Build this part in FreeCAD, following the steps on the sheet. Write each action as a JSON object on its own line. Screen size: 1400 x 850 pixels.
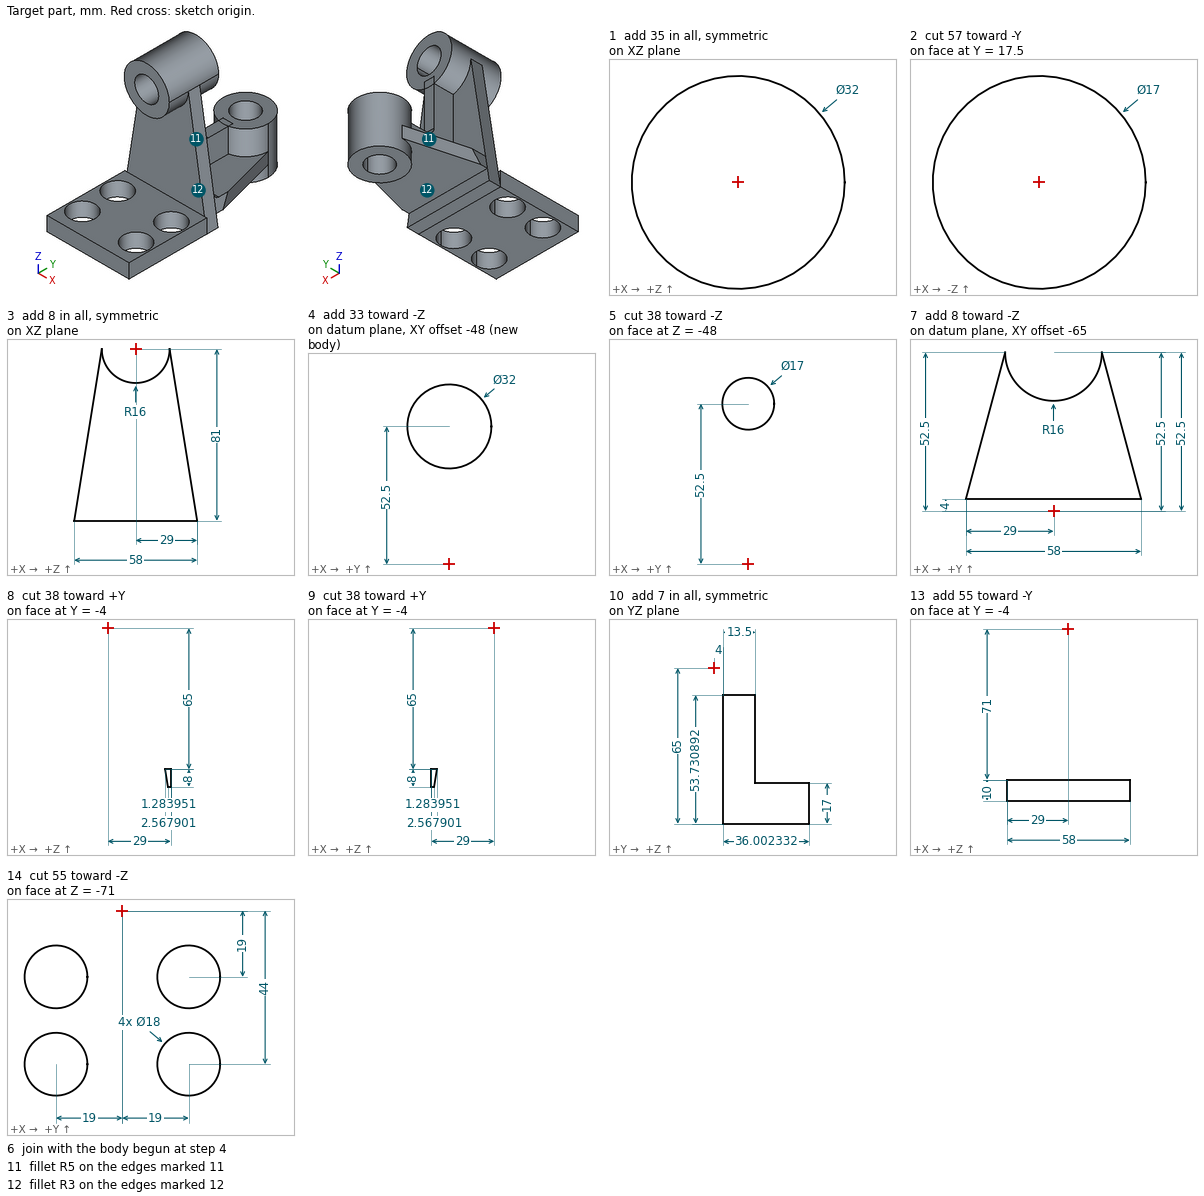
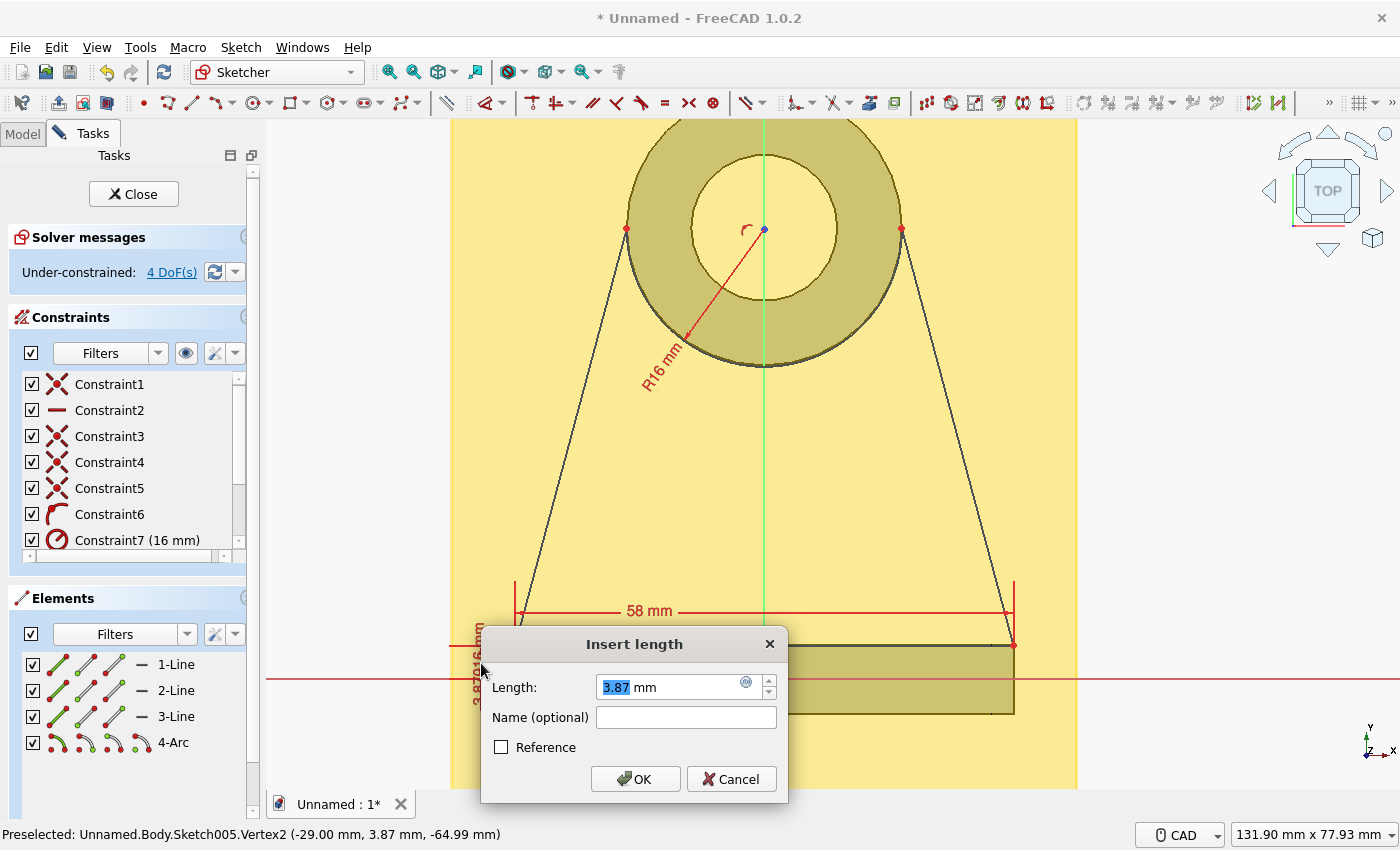
{"action": "type", "text": "4"}
{"action": "key", "text": "Return"}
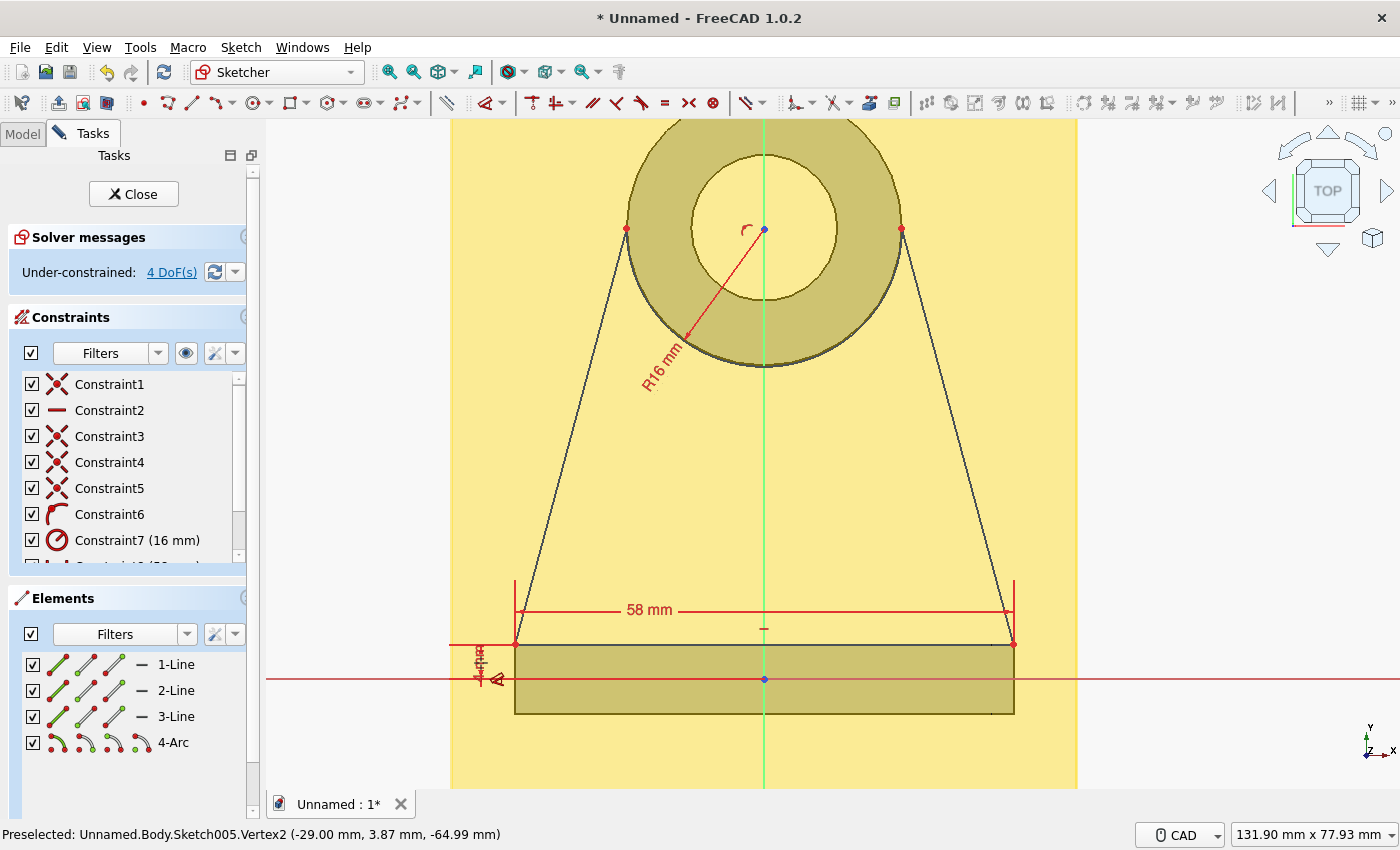
{"action": "left_click", "coordinate": [515, 645]}
{"action": "left_click", "coordinate": [640, 713]}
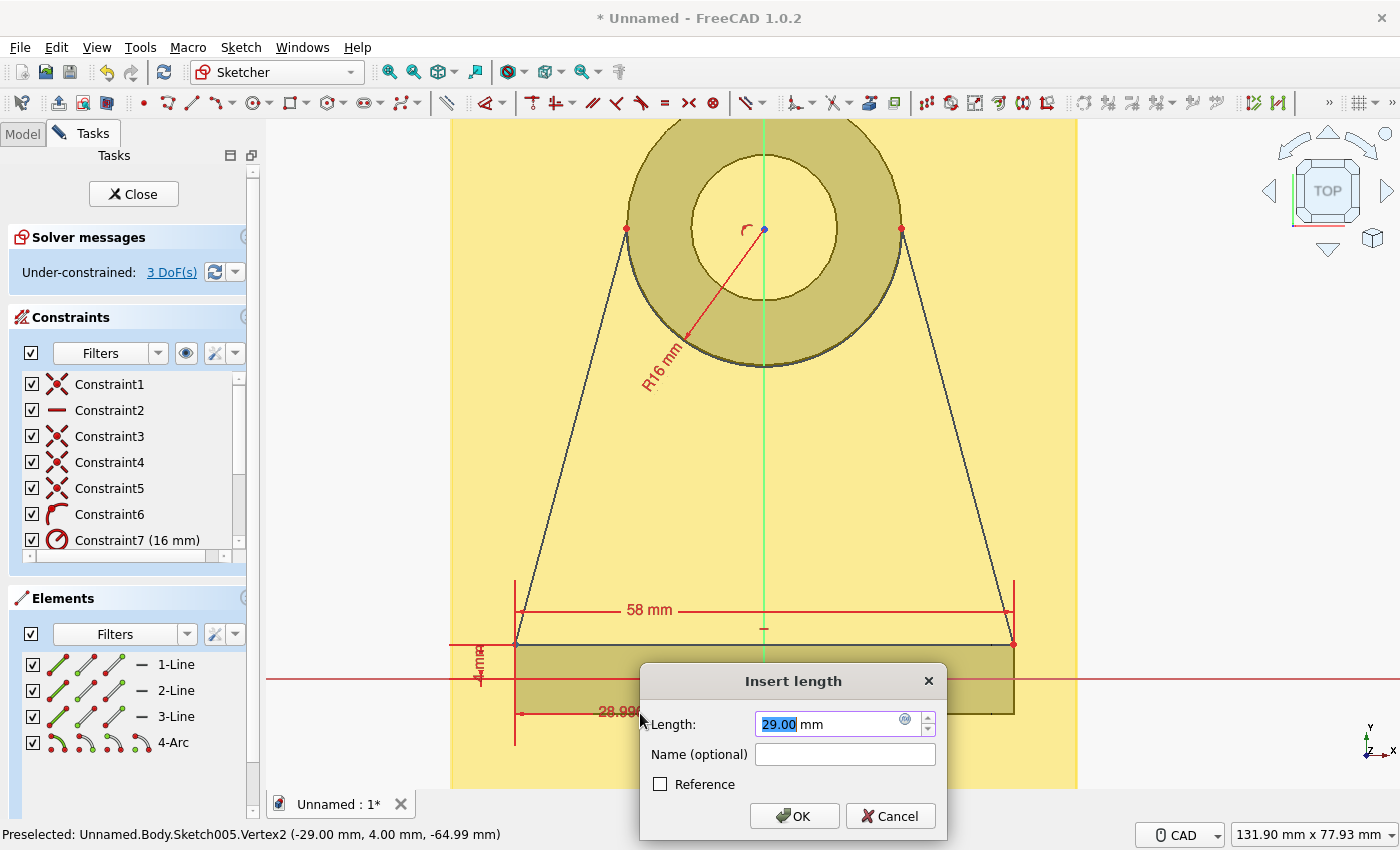
{"action": "type", "text": "29"}
{"action": "key", "text": "Return"}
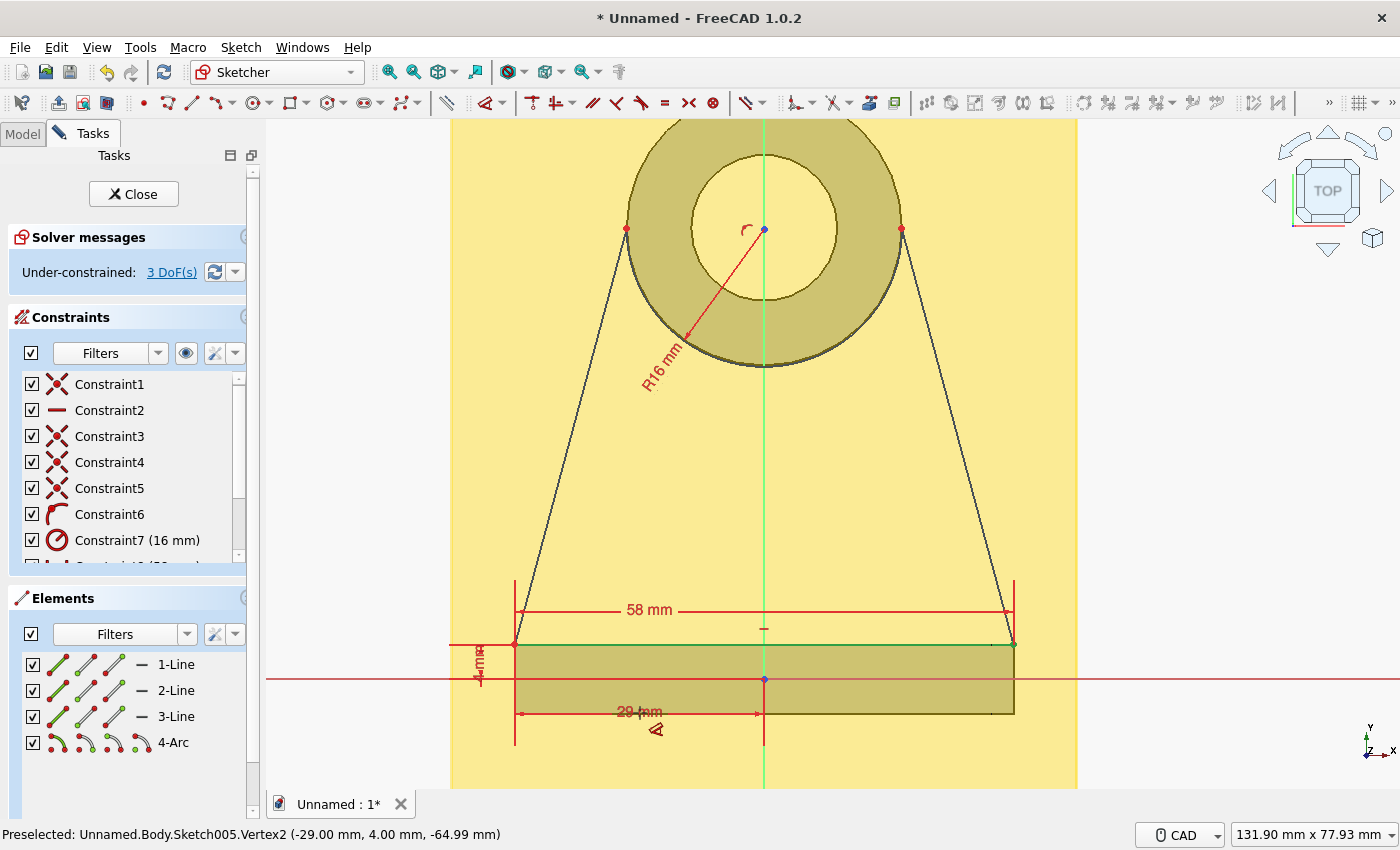
{"action": "left_click", "coordinate": [627, 229]}
{"action": "left_click", "coordinate": [593, 454]}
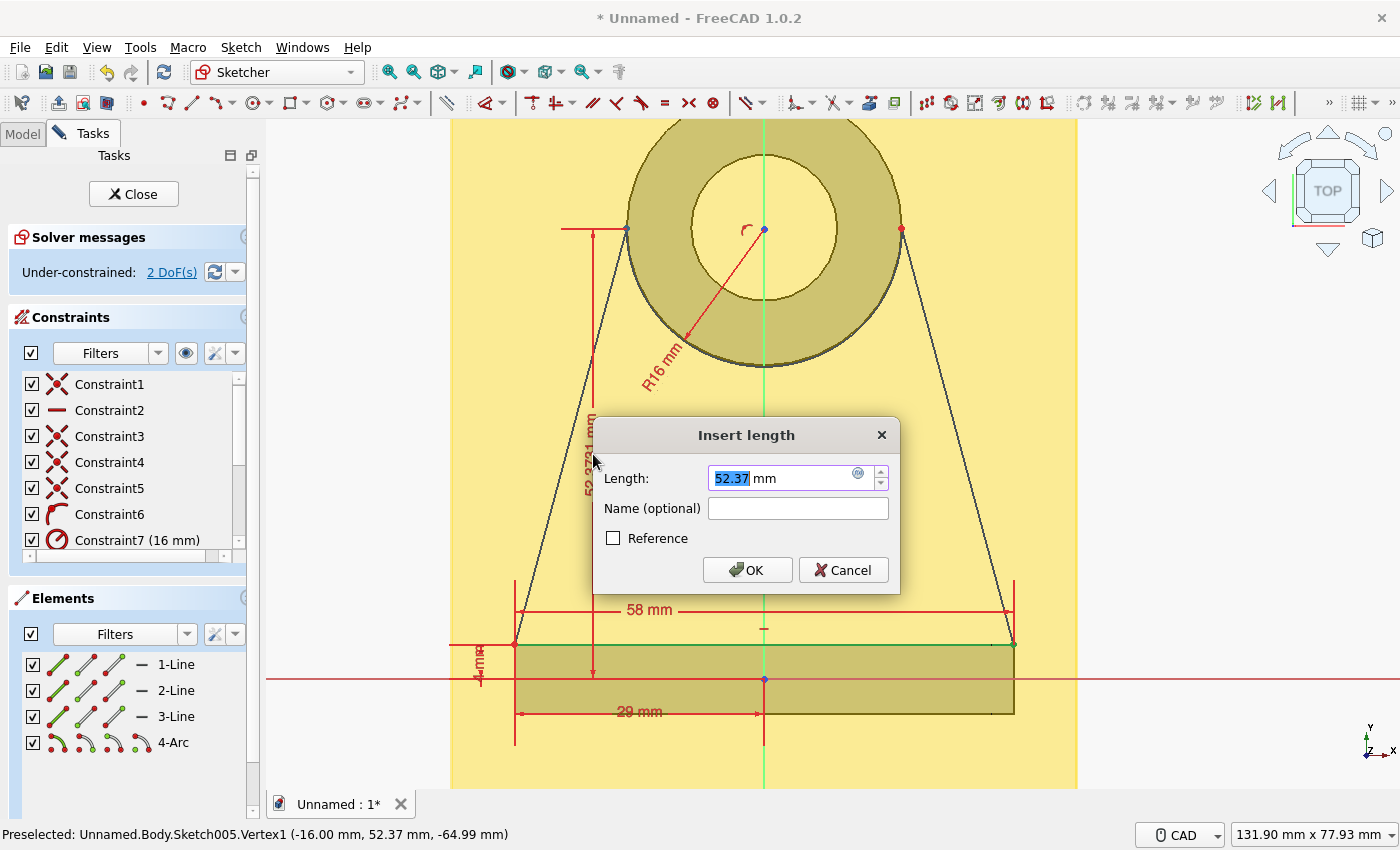
{"action": "type", "text": "52.5"}
{"action": "key", "text": "Return"}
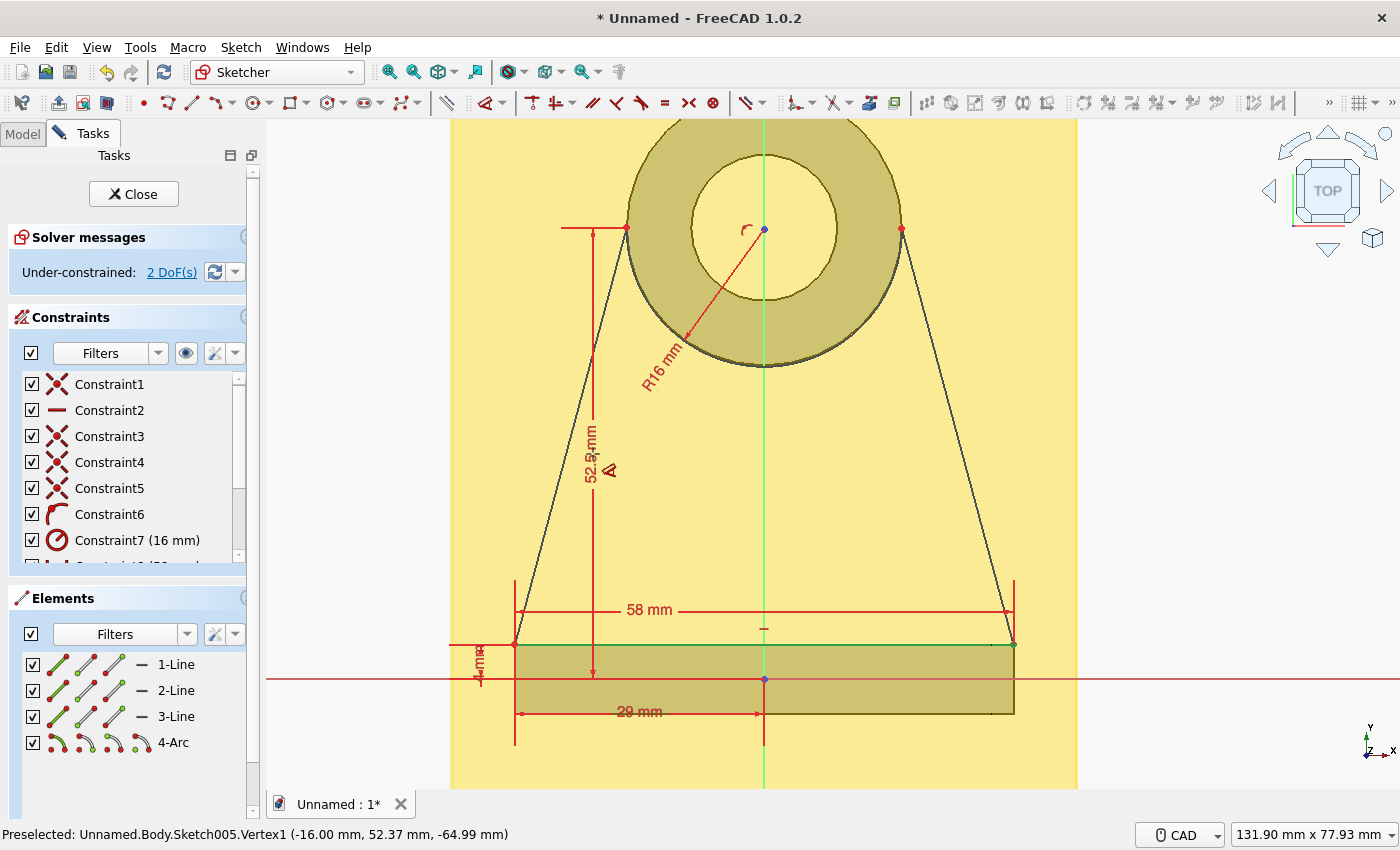
{"action": "left_click", "coordinate": [902, 229]}
{"action": "left_click", "coordinate": [936, 454]}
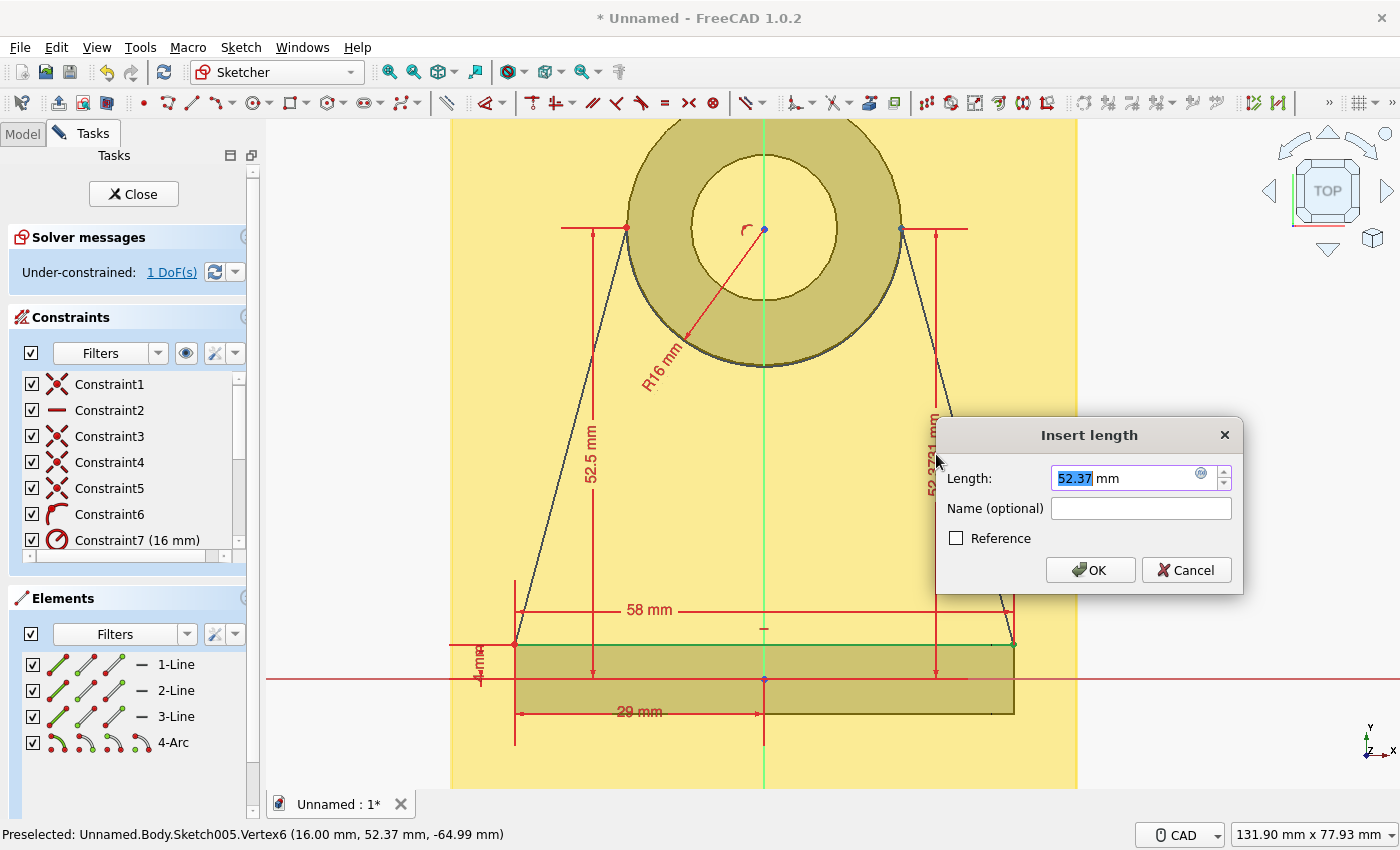
{"action": "type", "text": "52.5"}
{"action": "key", "text": "Return"}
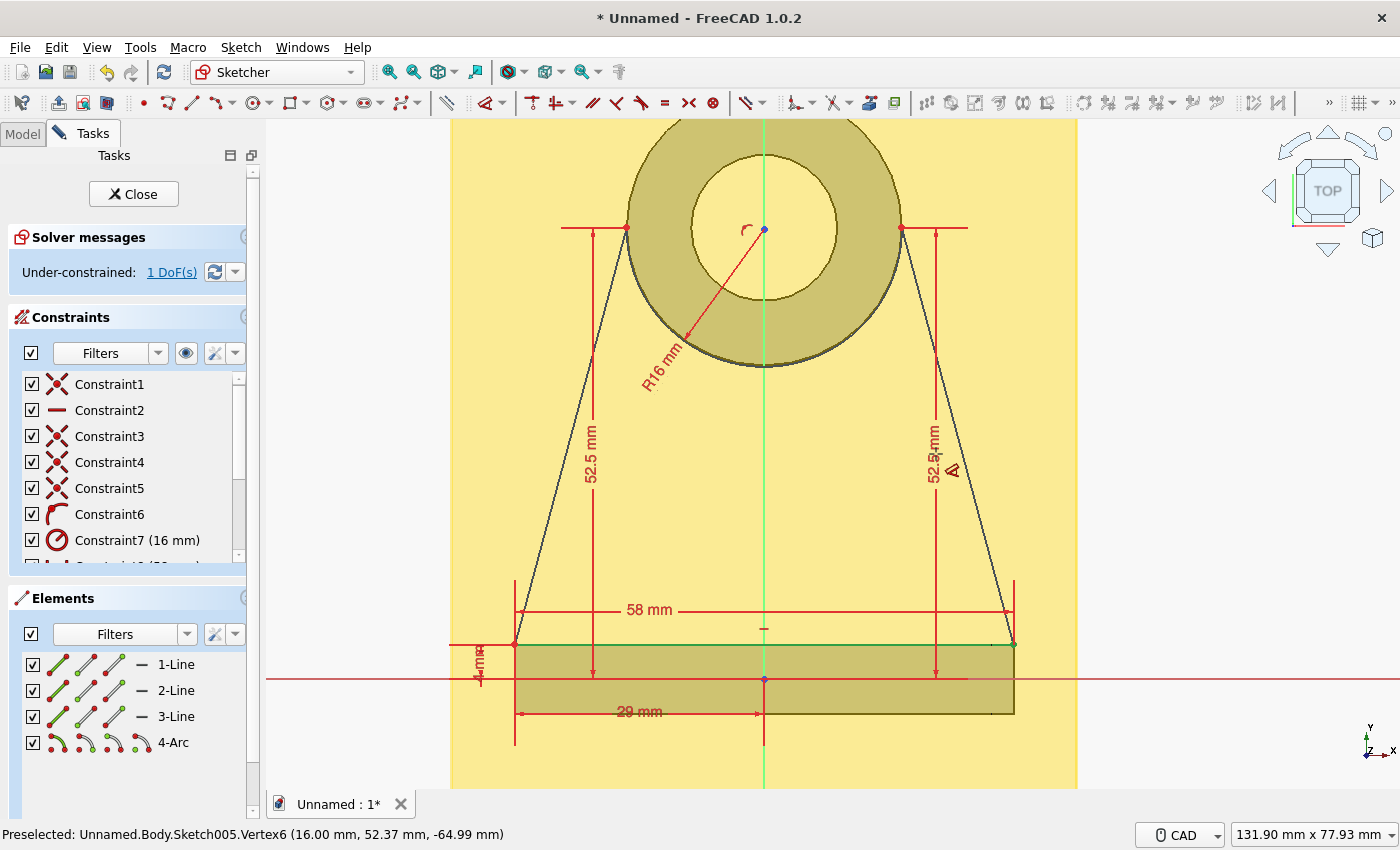
{"action": "left_click", "coordinate": [764, 229]}
{"action": "left_click", "coordinate": [798, 454]}